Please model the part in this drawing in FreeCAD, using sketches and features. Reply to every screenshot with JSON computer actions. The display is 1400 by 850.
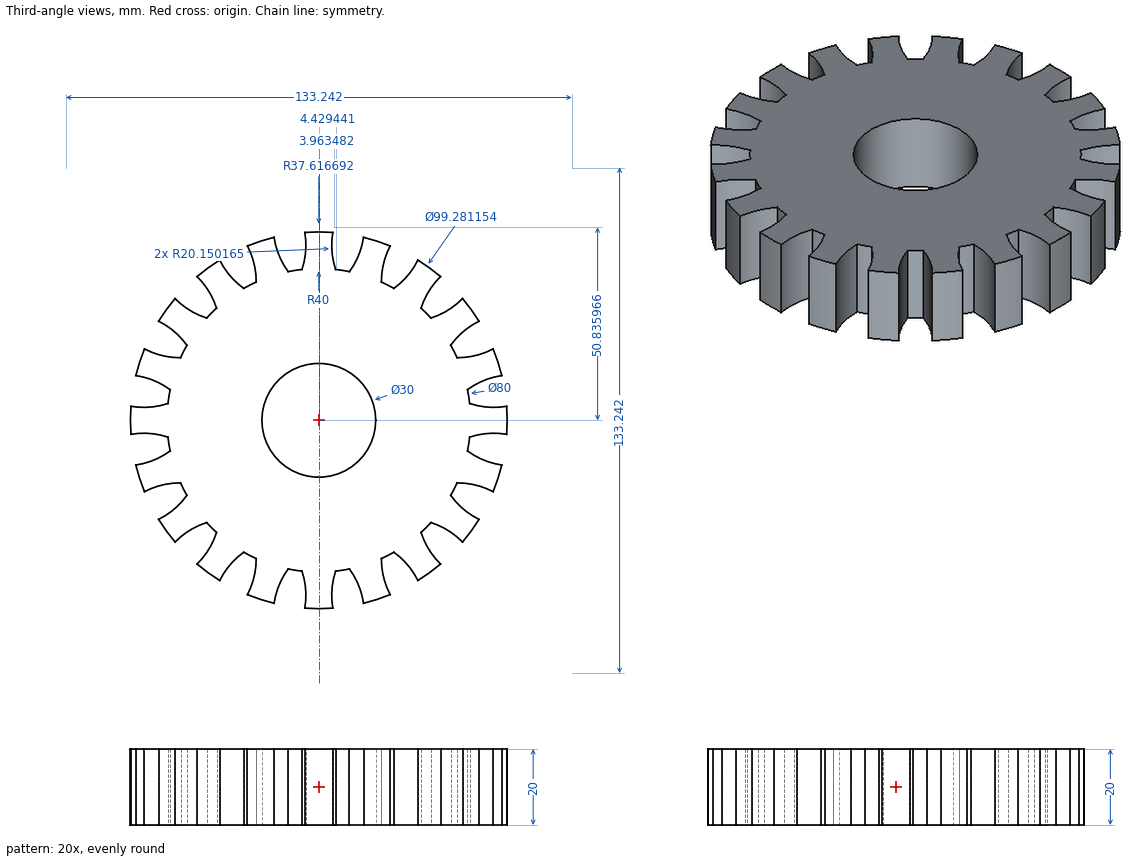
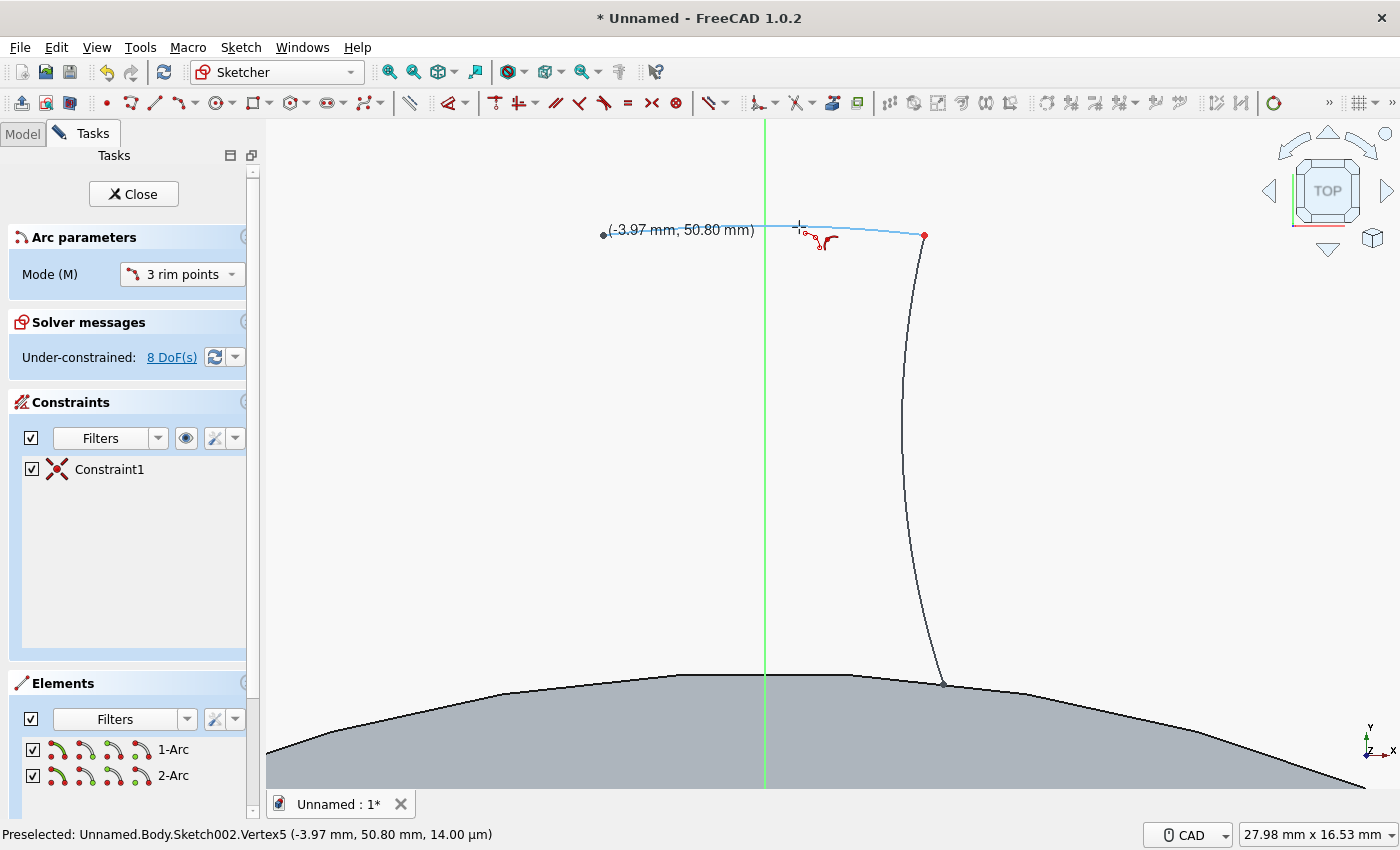
{"action": "left_click", "coordinate": [585, 683]}
{"action": "left_click", "coordinate": [626, 460]}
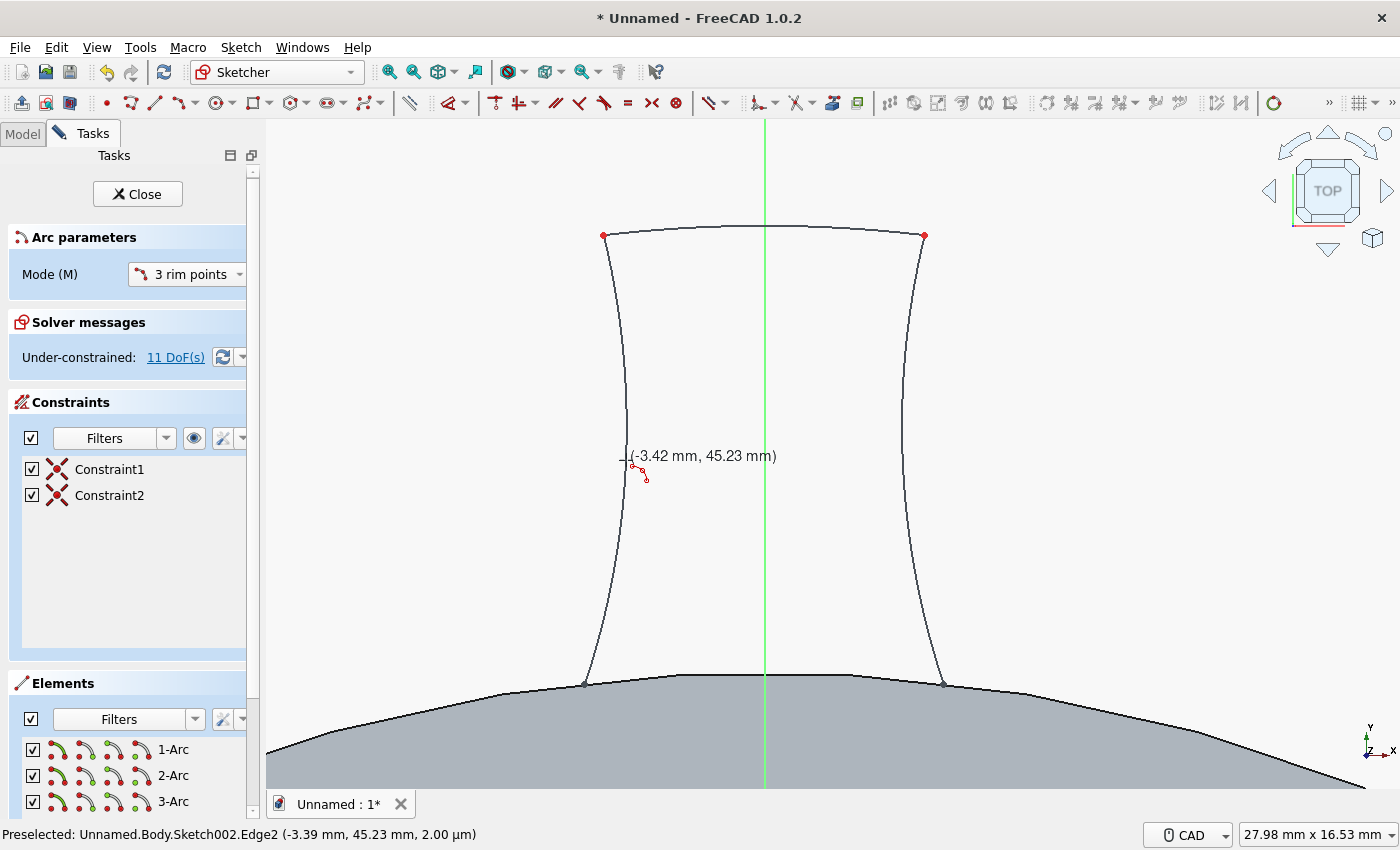
{"action": "left_click", "coordinate": [585, 684]}
{"action": "left_click", "coordinate": [944, 684]}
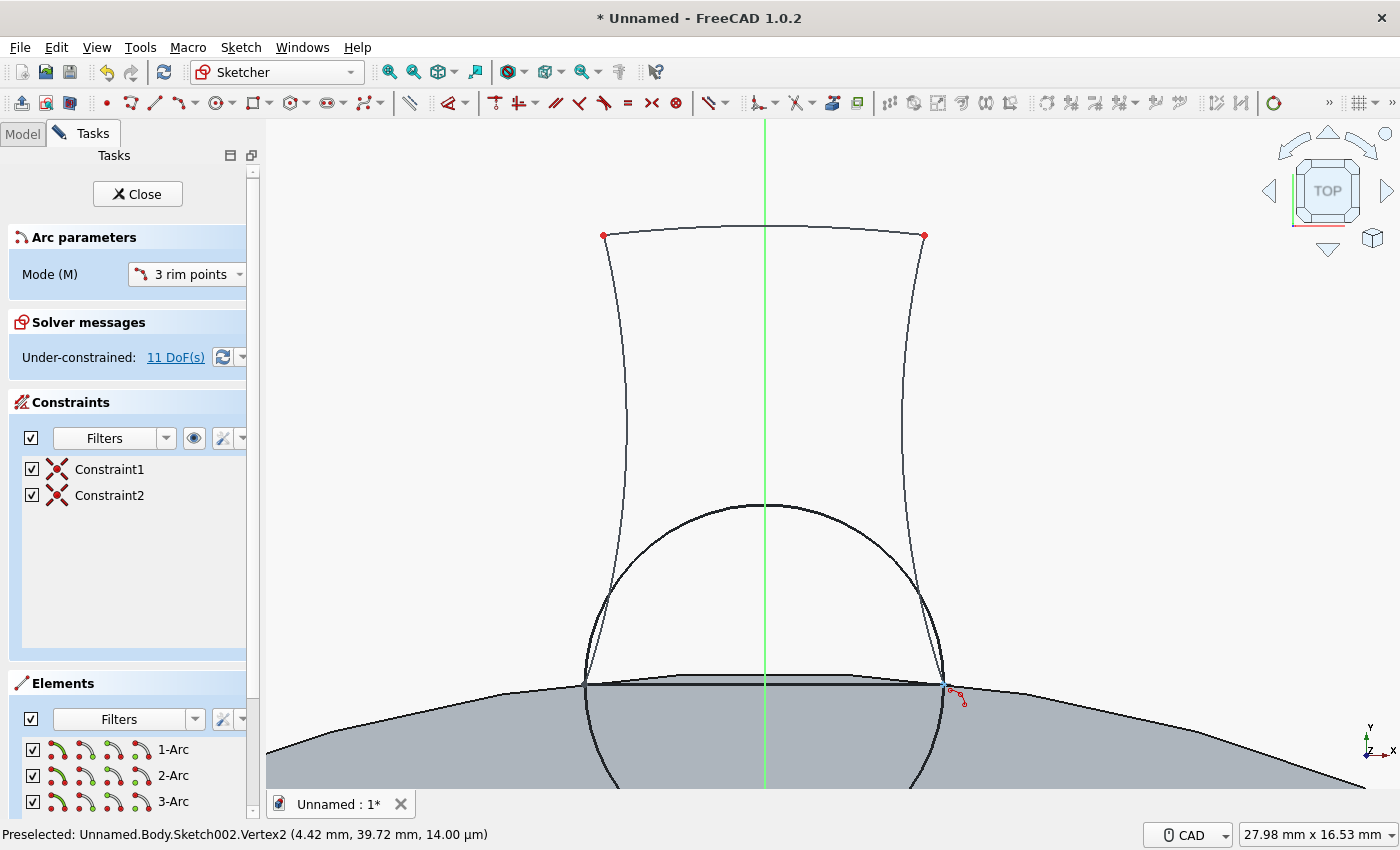
{"action": "scroll", "coordinate": [801, 673], "scroll_direction": "up", "scroll_amount": 3}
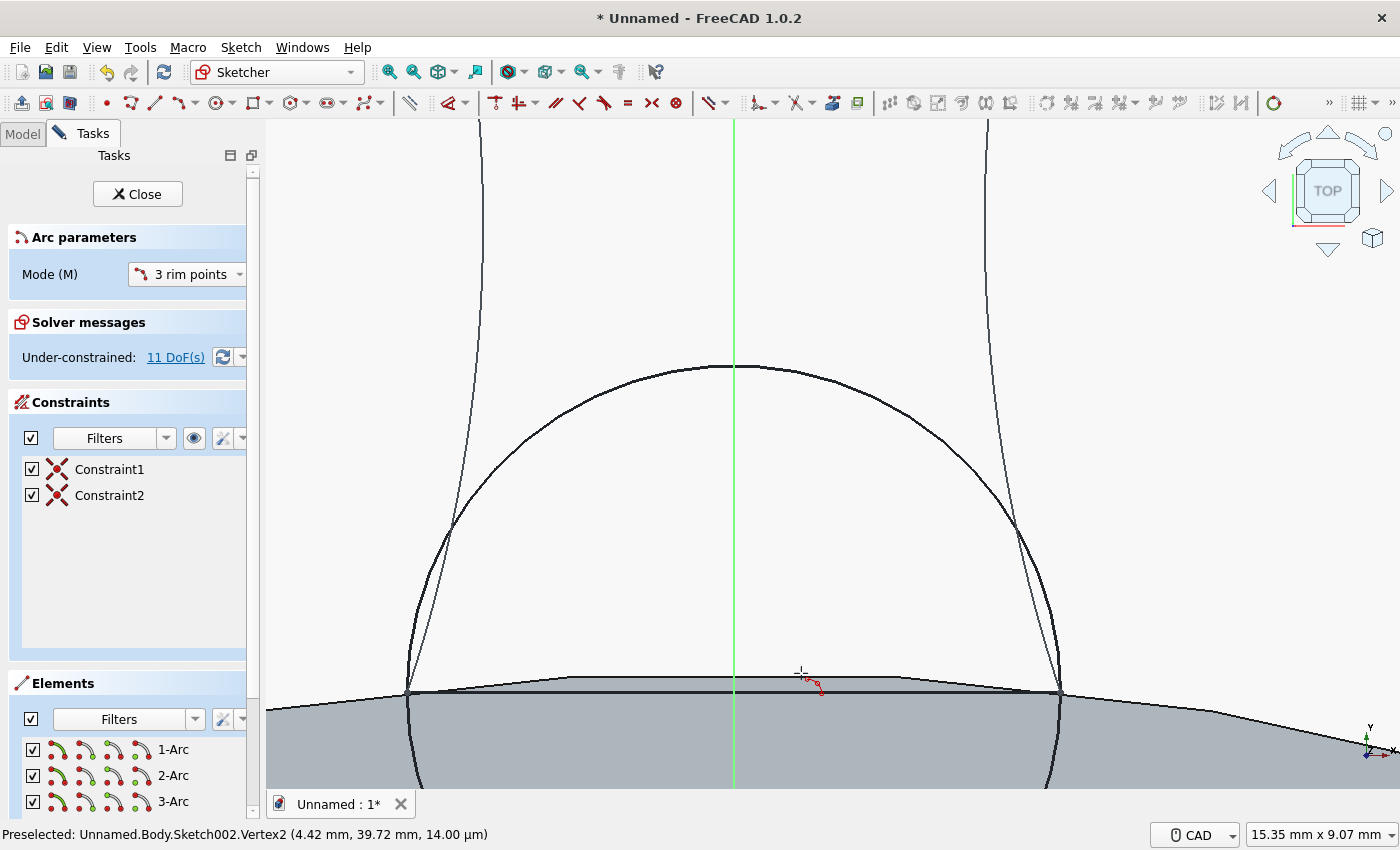
{"action": "left_click", "coordinate": [800, 673]}
{"action": "key", "text": "Escape"}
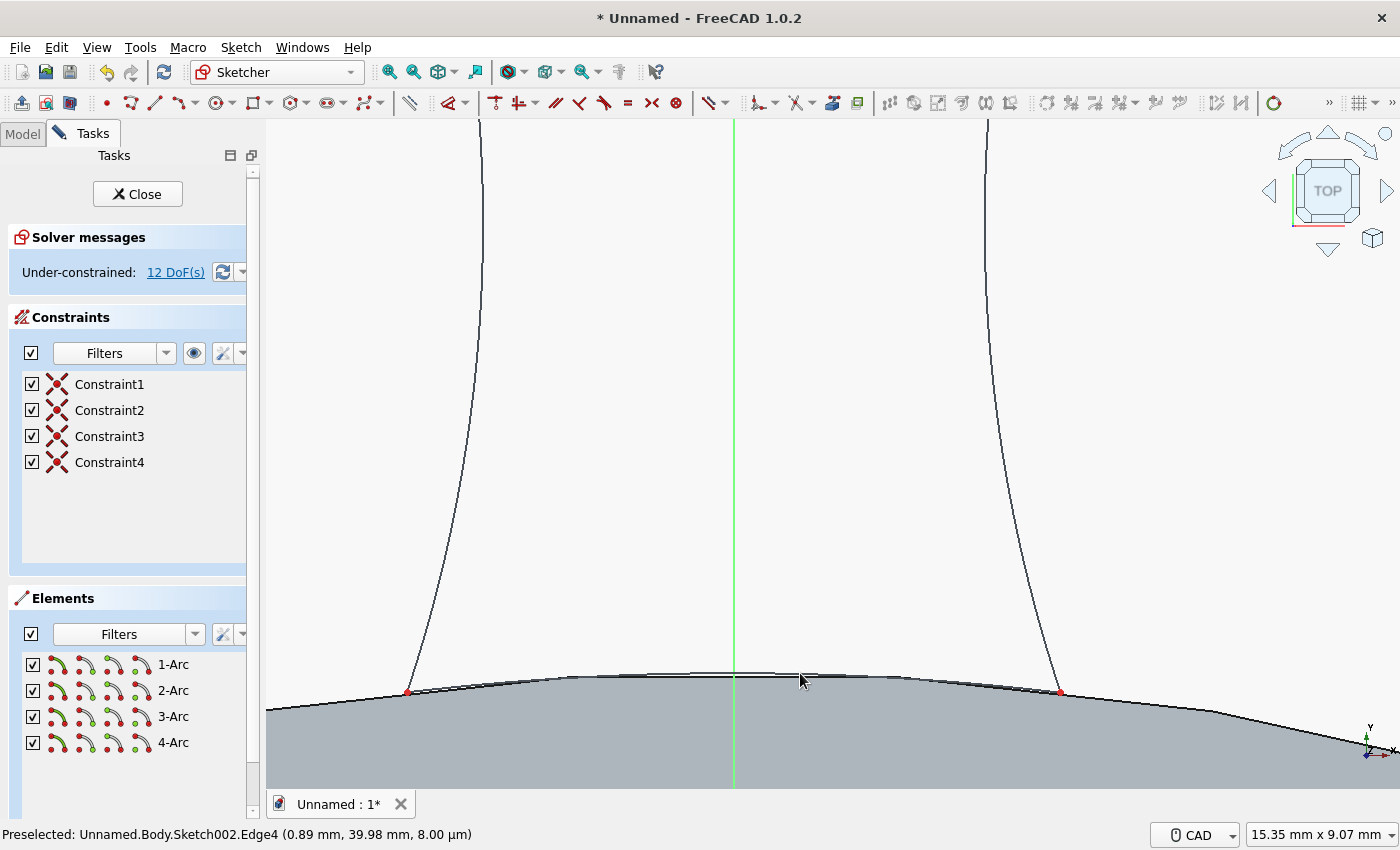
{"action": "scroll", "coordinate": [801, 673], "scroll_direction": "down", "scroll_amount": 3}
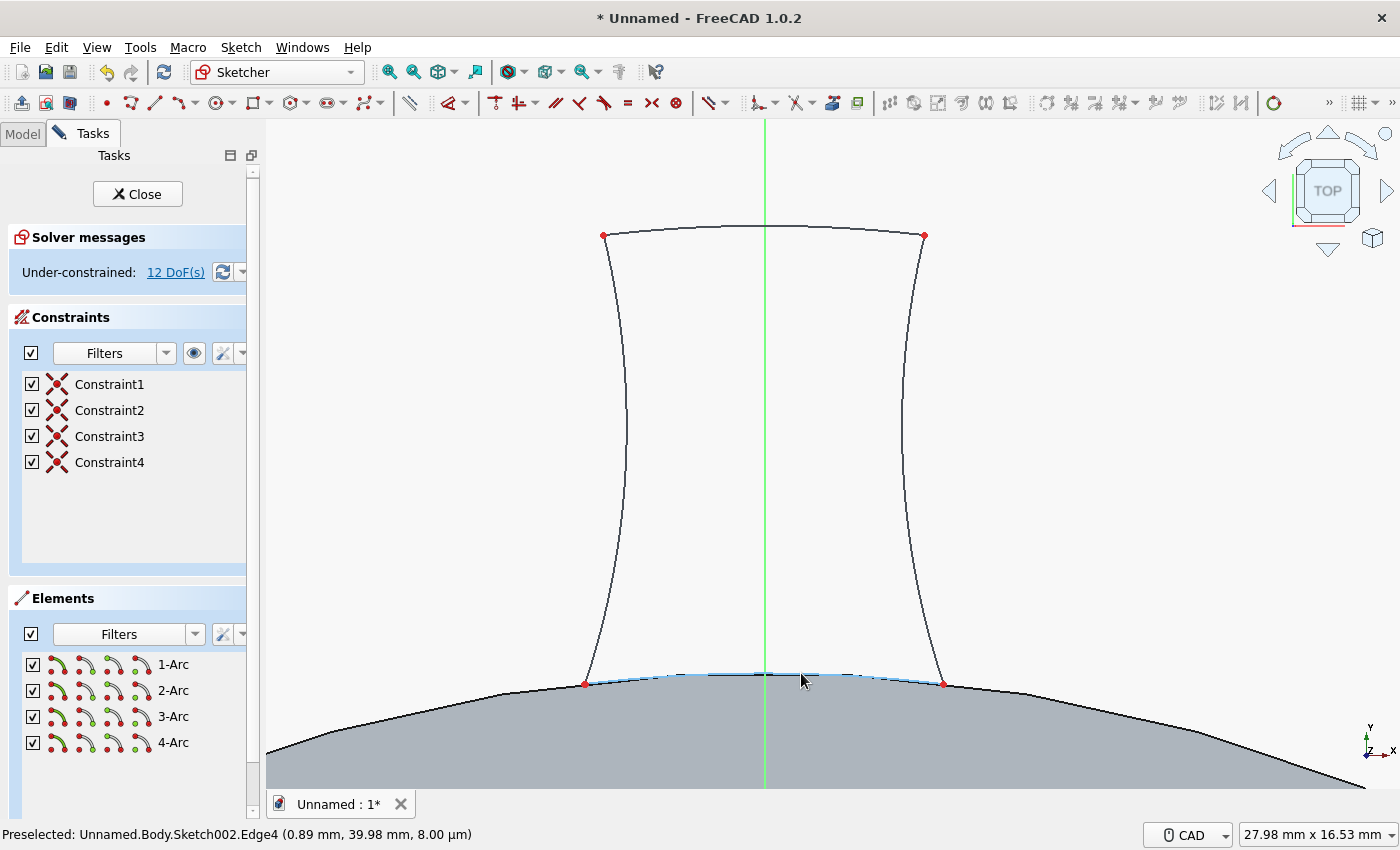
{"action": "scroll", "coordinate": [764, 257], "scroll_direction": "down", "scroll_amount": 8}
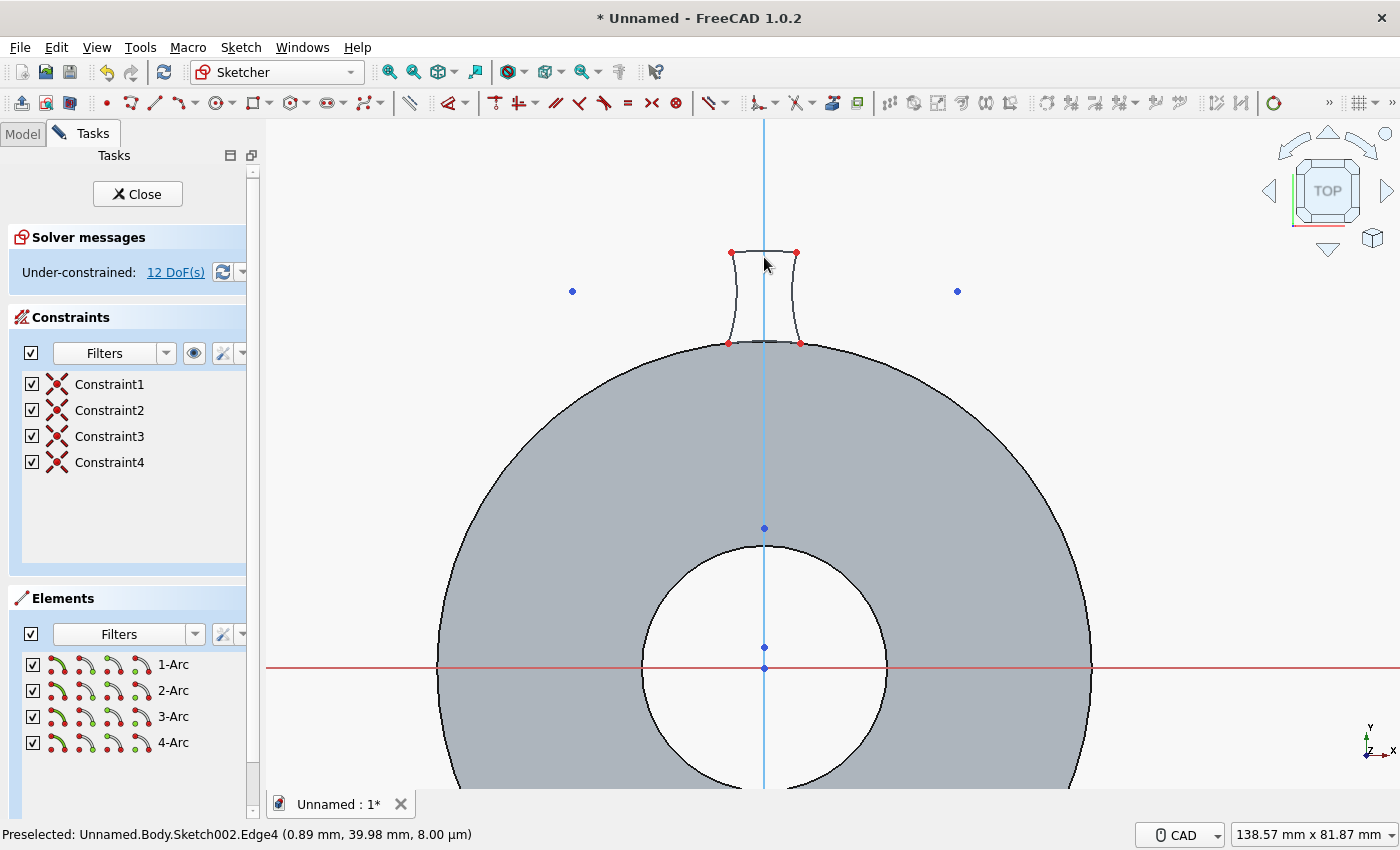
{"action": "left_click_drag", "start_coordinate": [754, 638], "coordinate": [774, 678]}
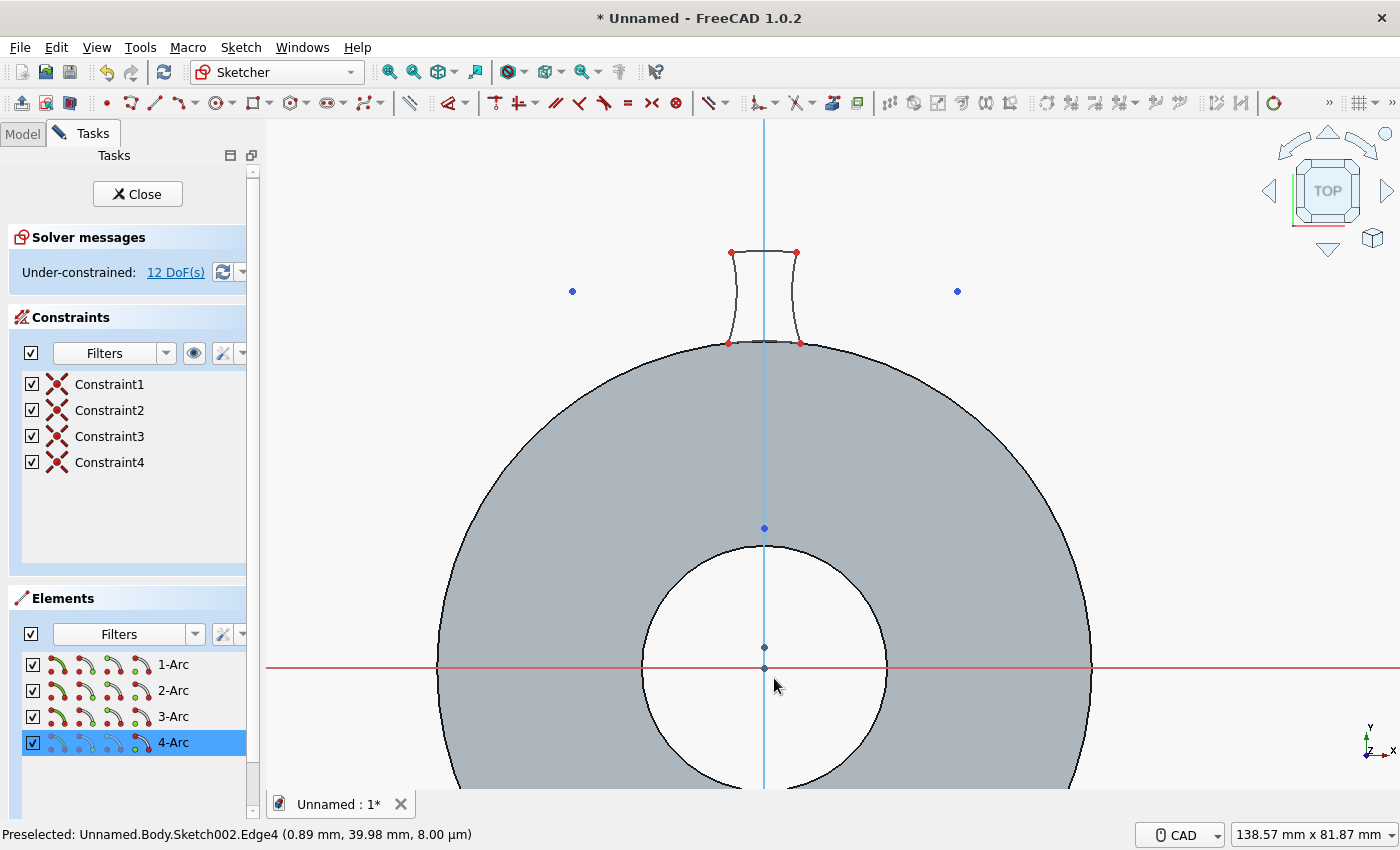
{"action": "key", "text": "c"}